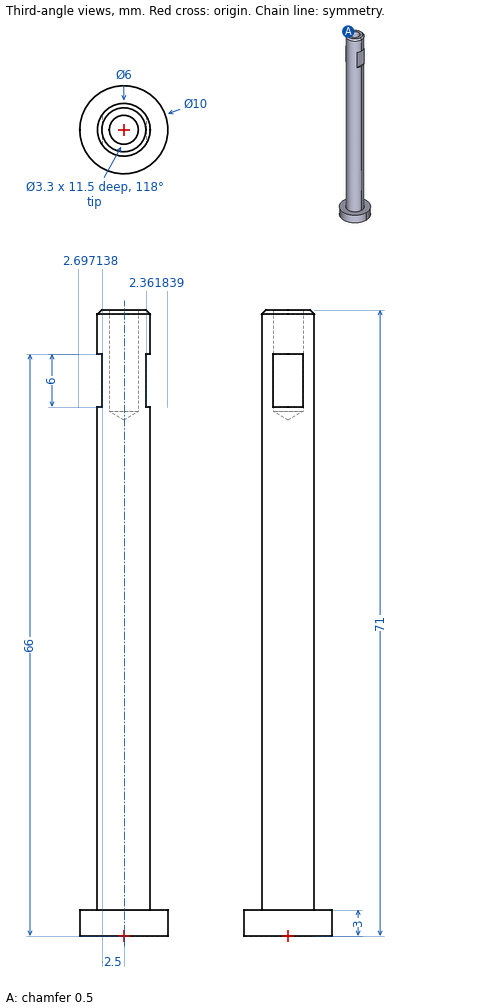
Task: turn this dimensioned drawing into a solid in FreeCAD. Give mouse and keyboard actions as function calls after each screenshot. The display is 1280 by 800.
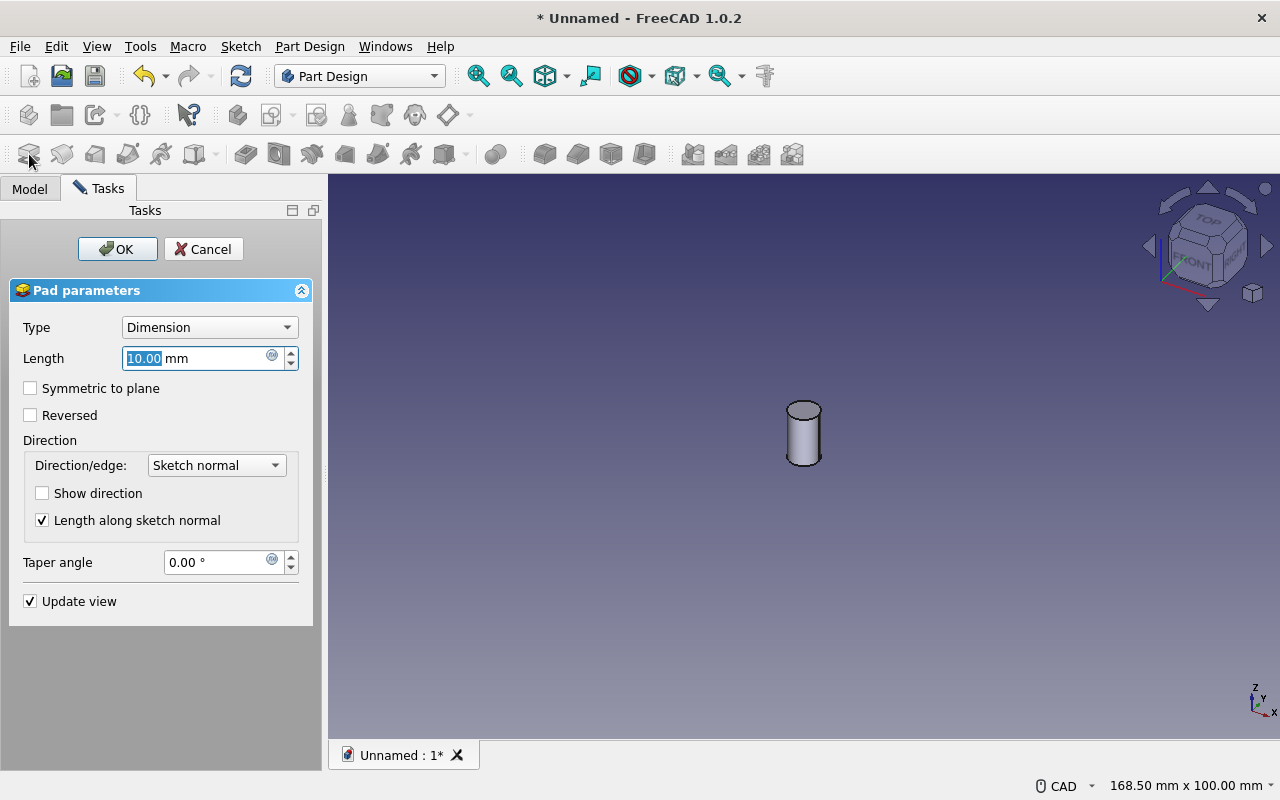
text(71)
key(Tab)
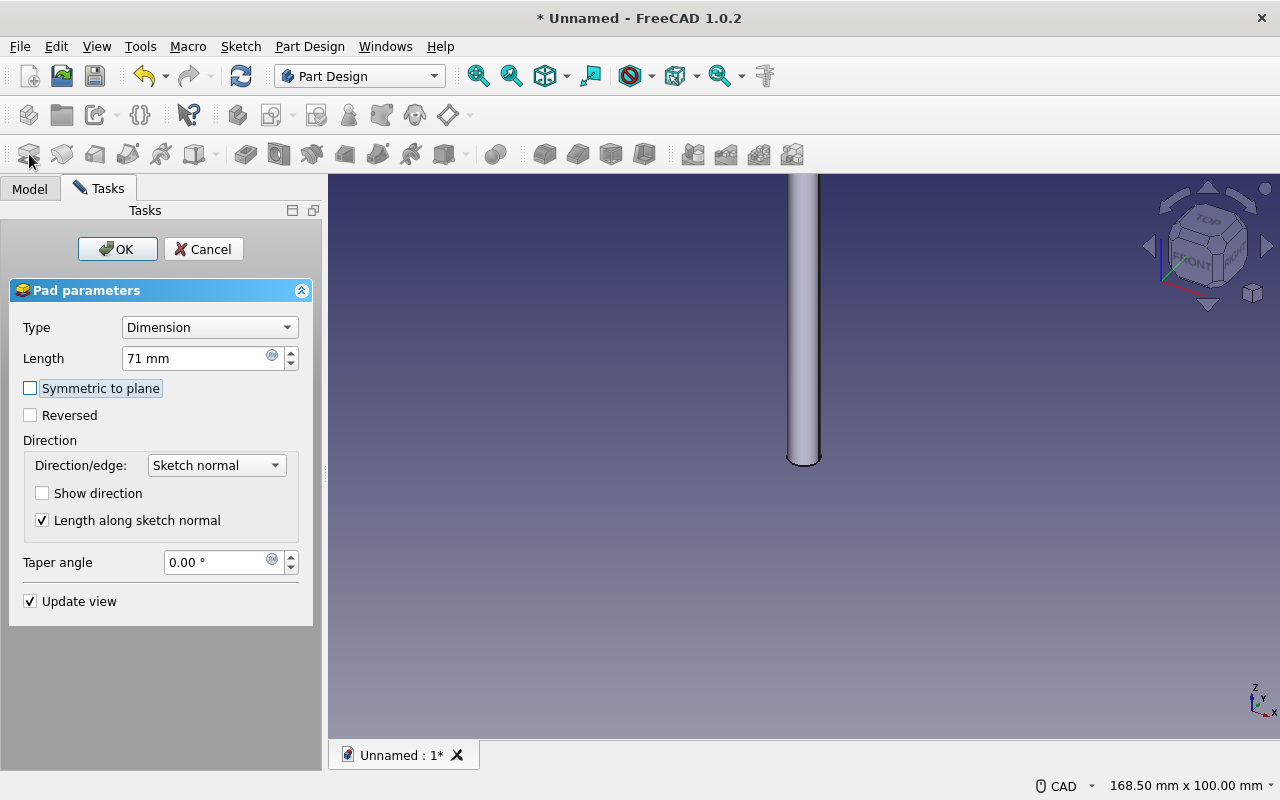
click(118, 249)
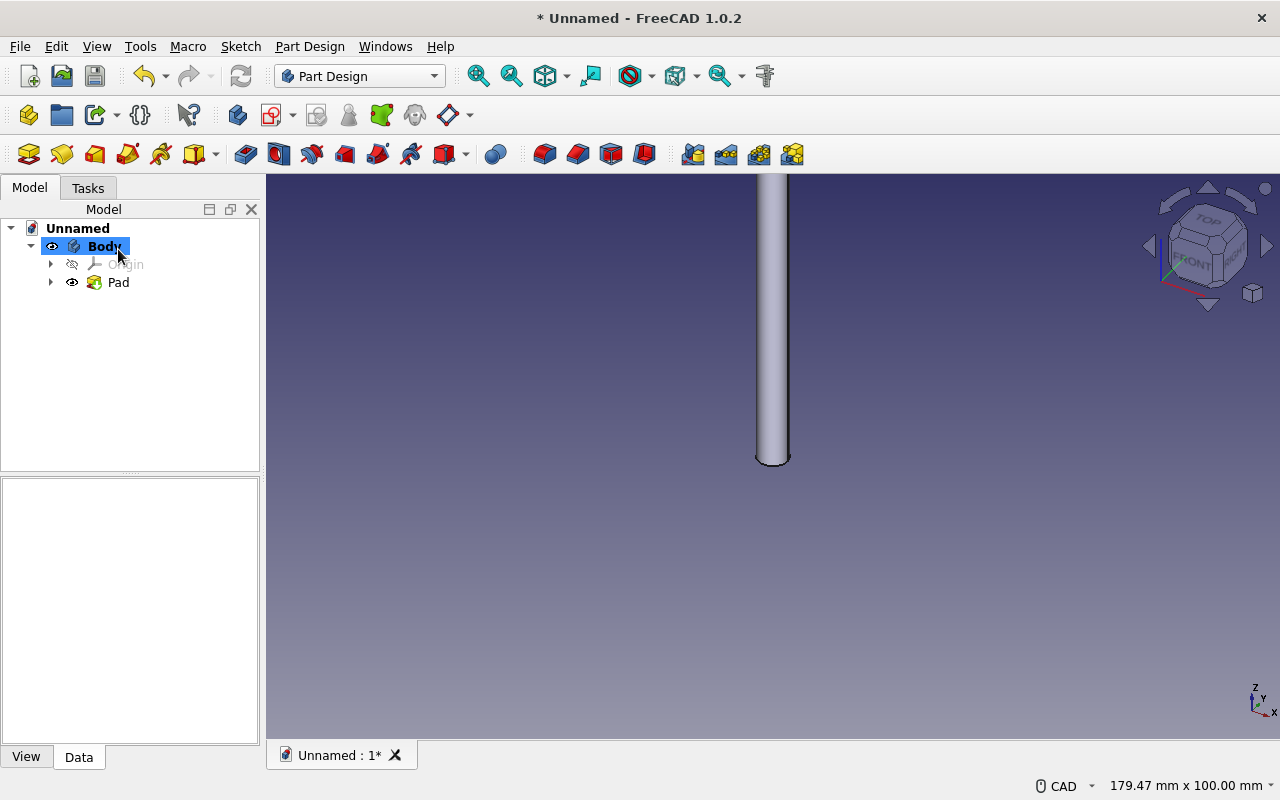
key(v)
key(f)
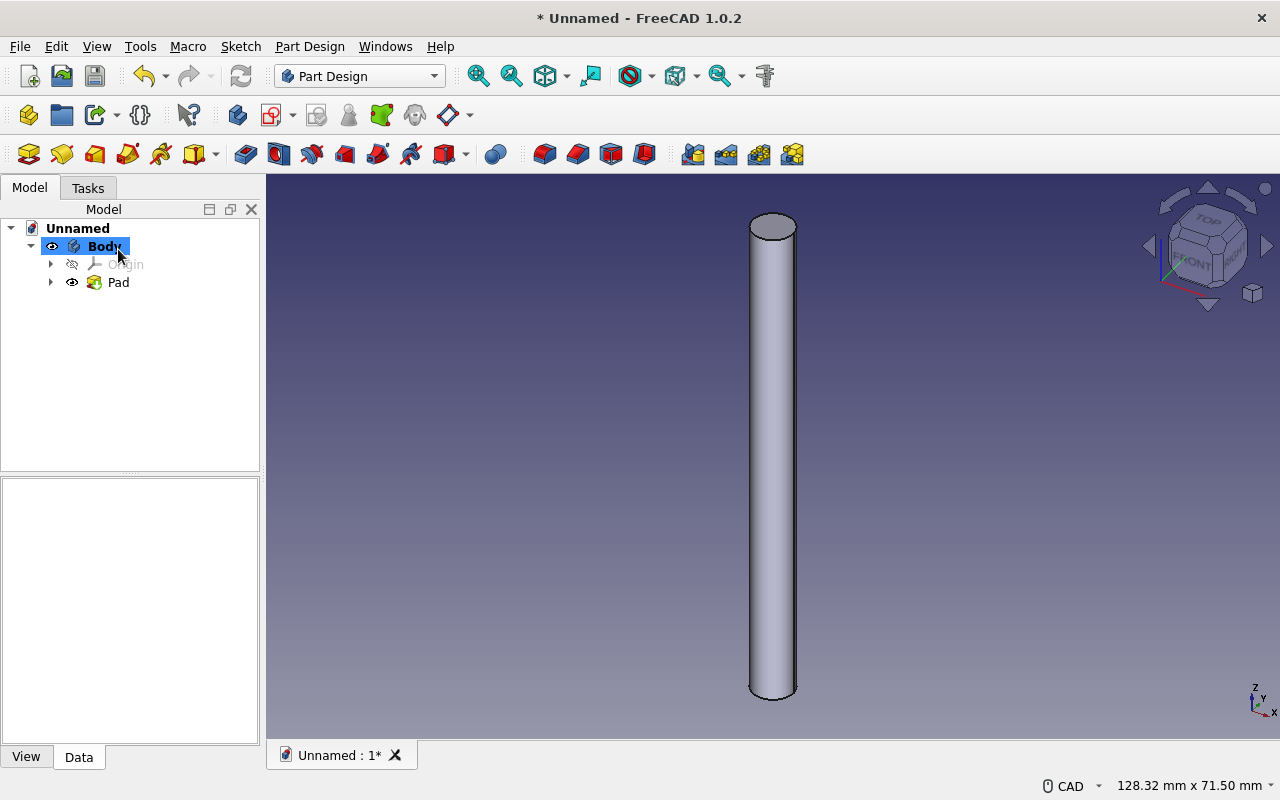
click(773, 226)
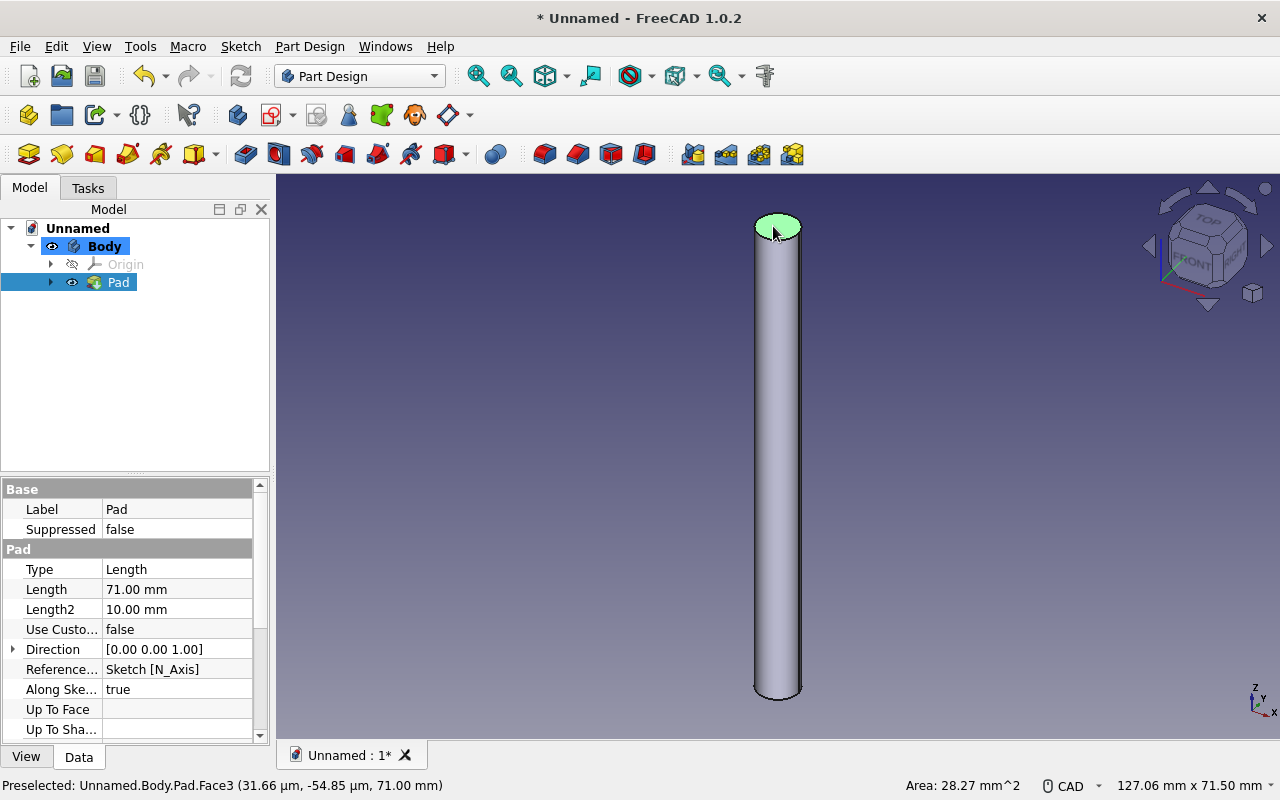
click(270, 116)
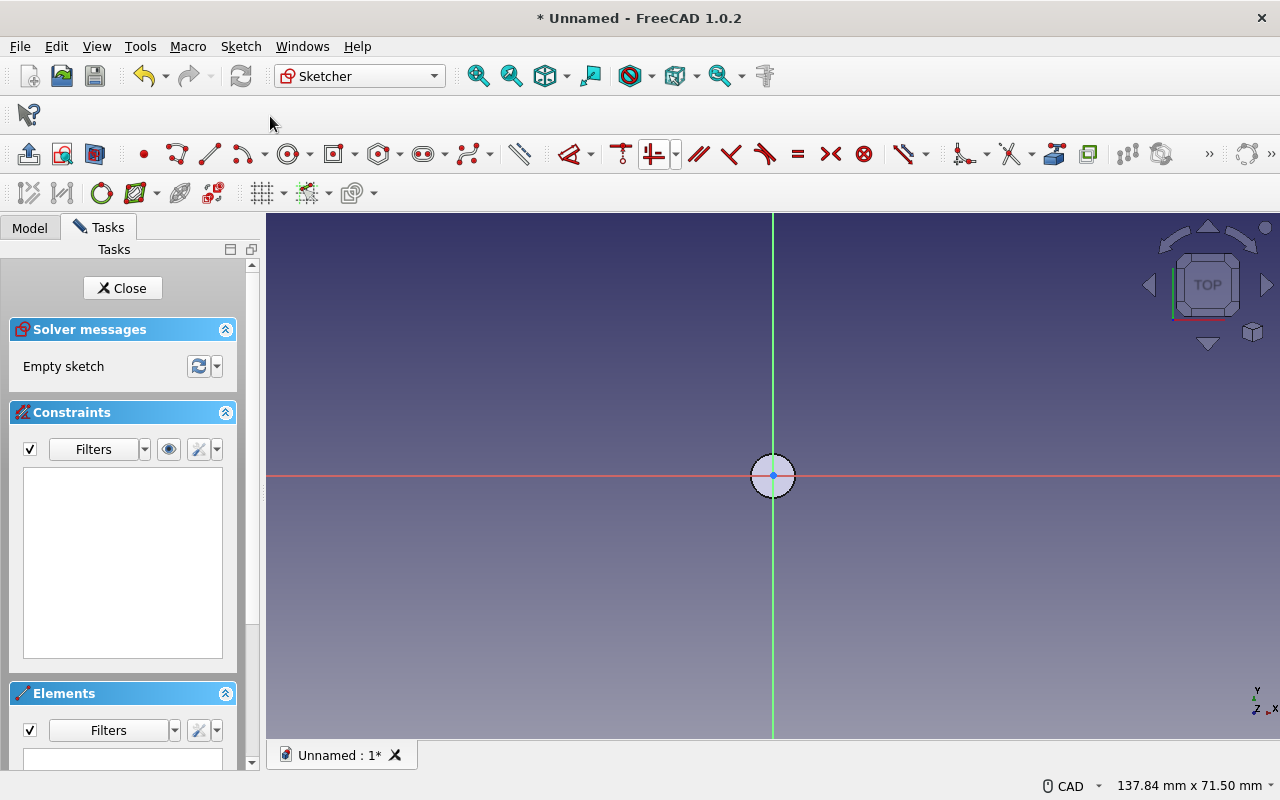
scroll(778, 476, up, 13)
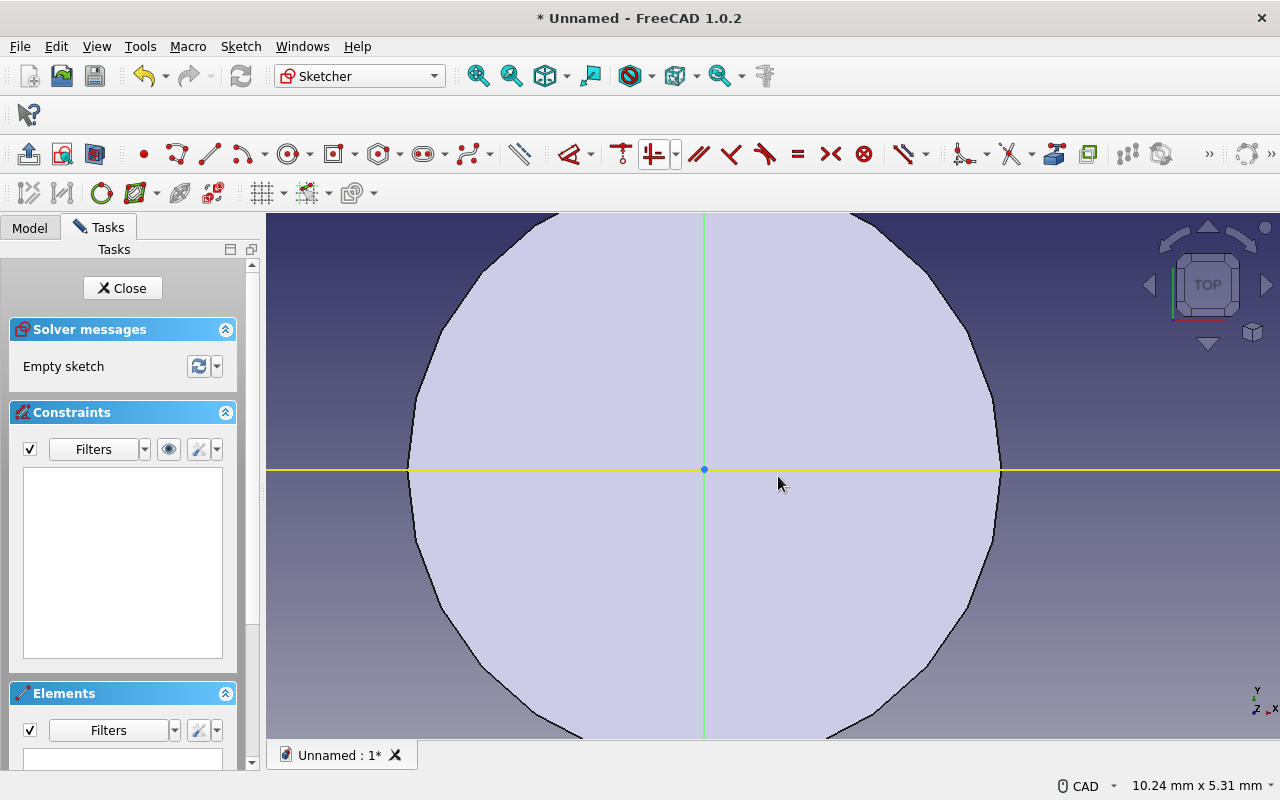
key(g)
key(c)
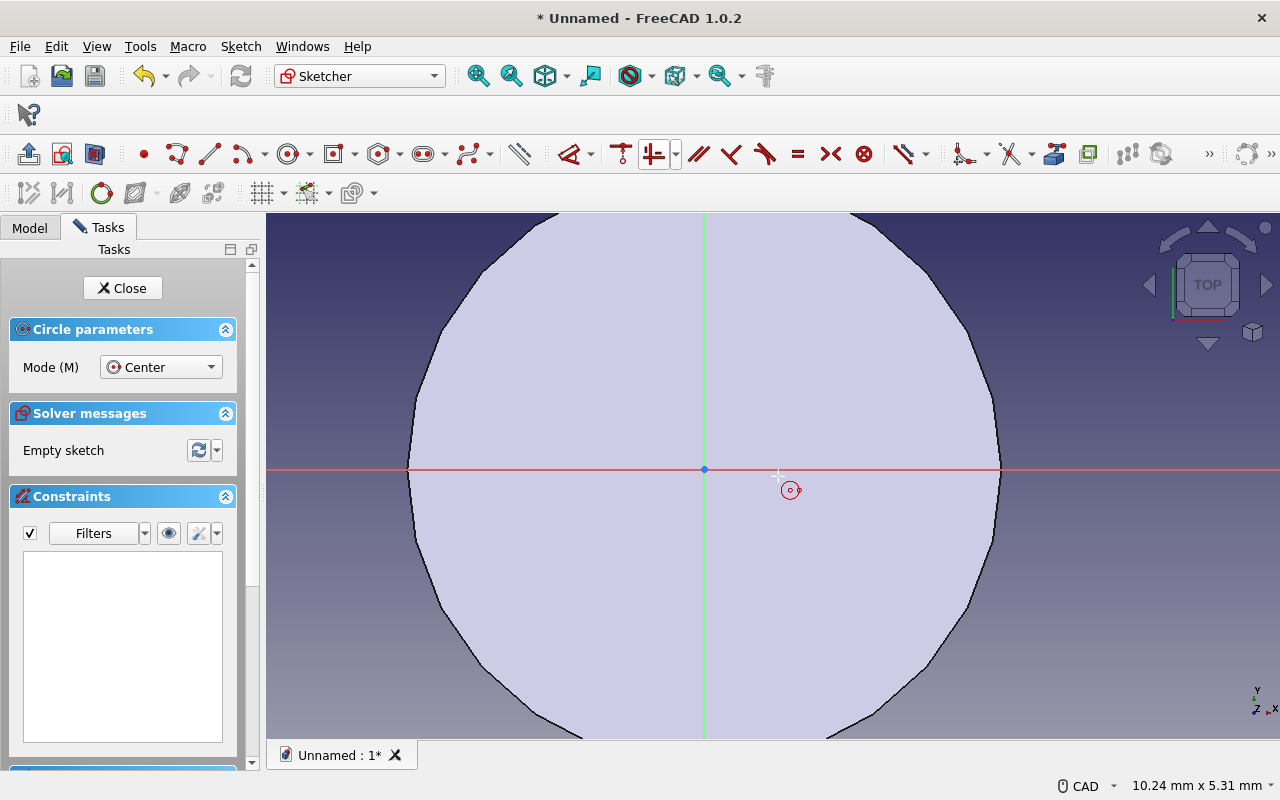
click(704, 470)
move(820, 354)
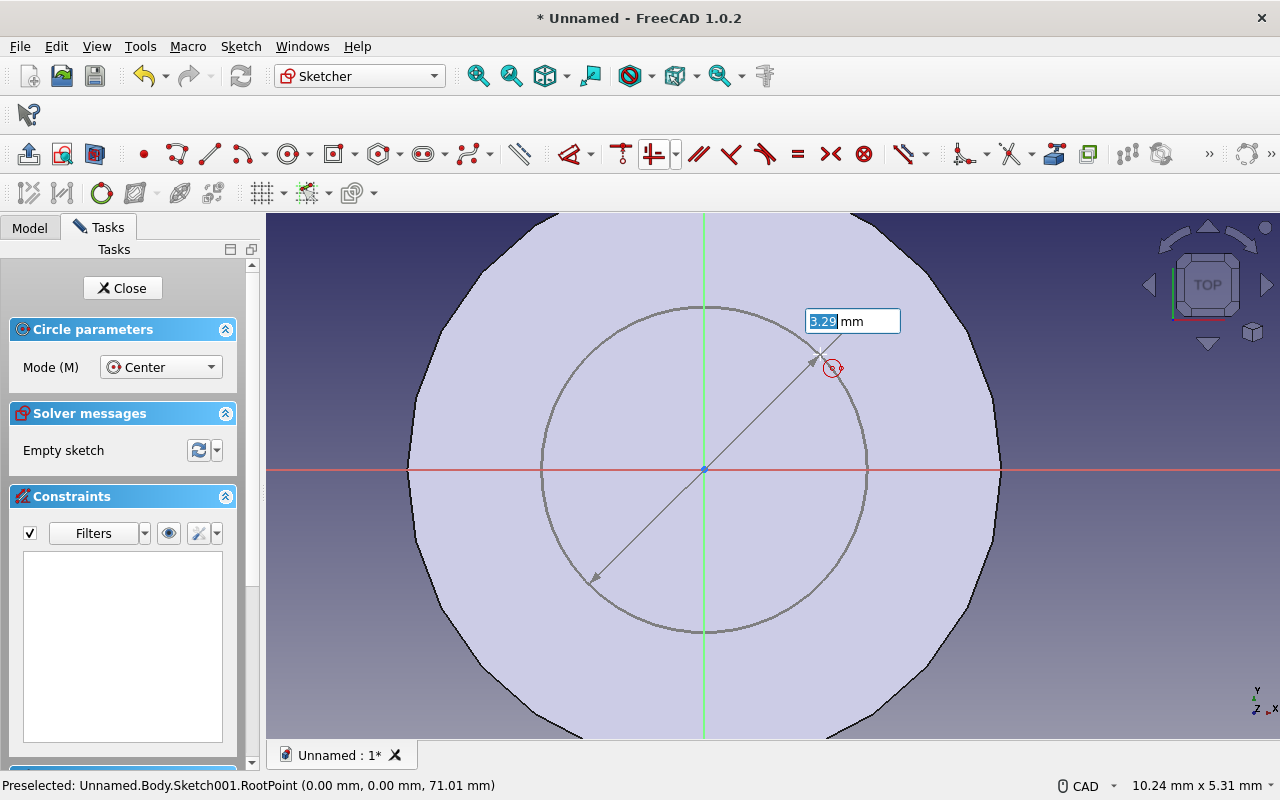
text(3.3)
key(Return)
key(Escape)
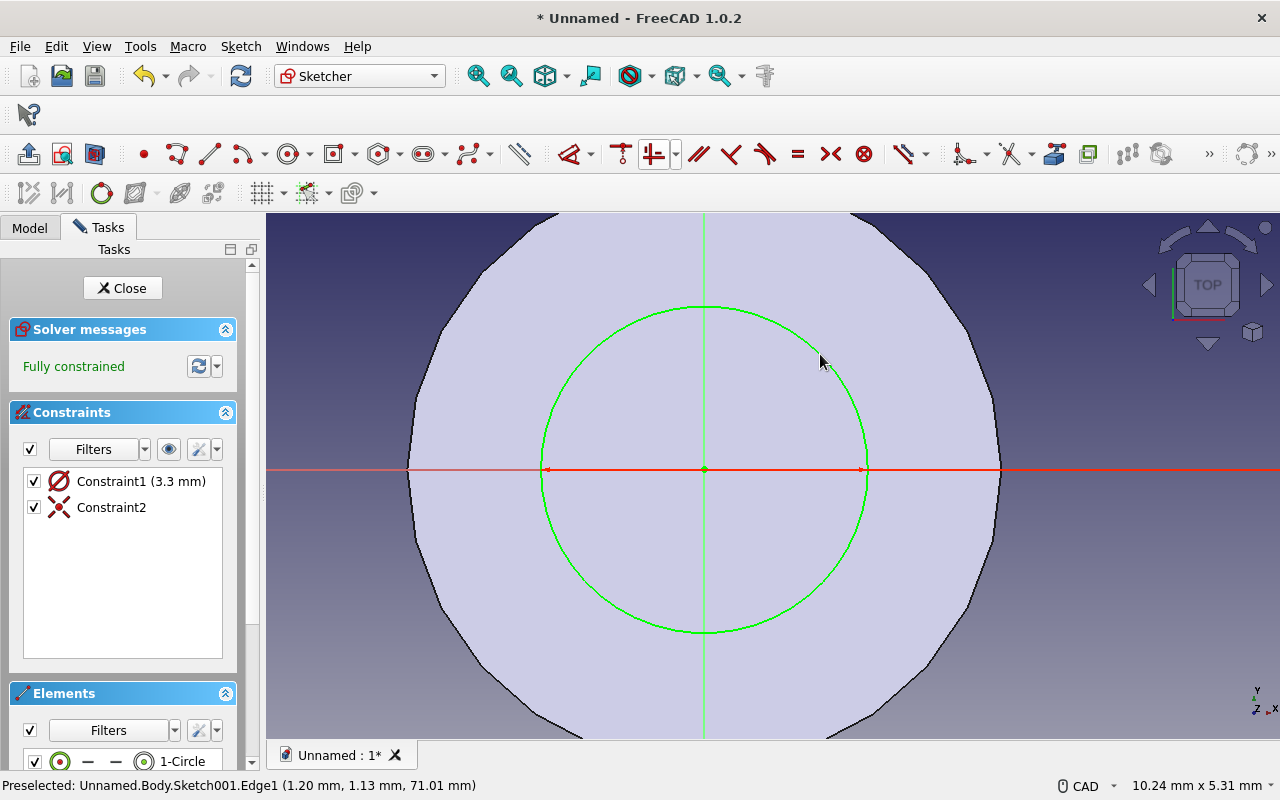
click(123, 288)